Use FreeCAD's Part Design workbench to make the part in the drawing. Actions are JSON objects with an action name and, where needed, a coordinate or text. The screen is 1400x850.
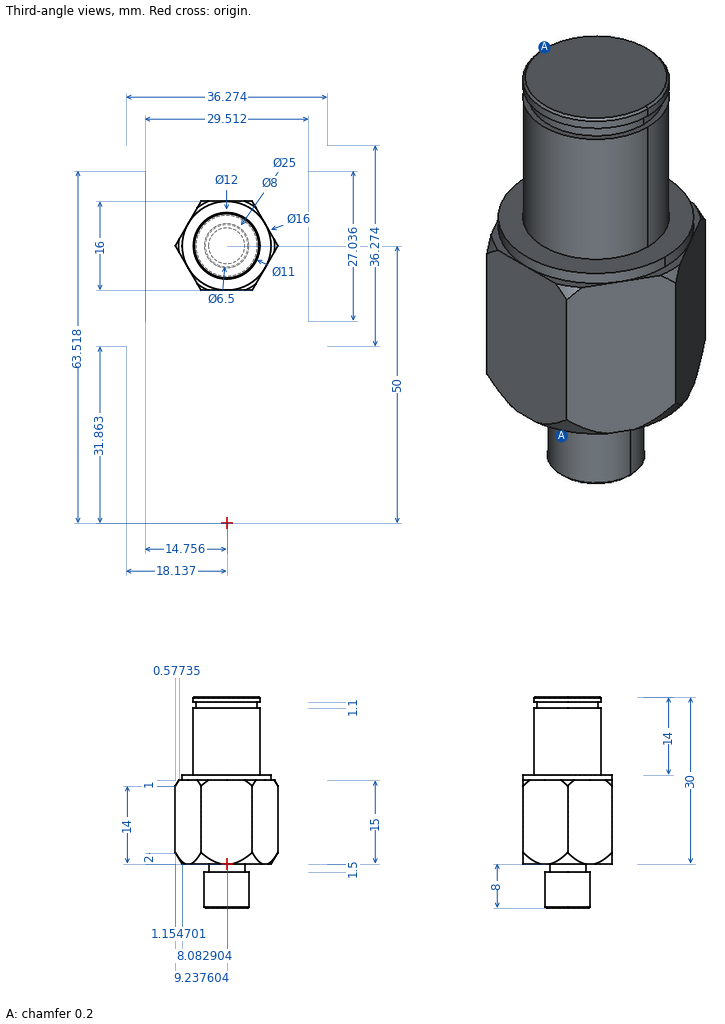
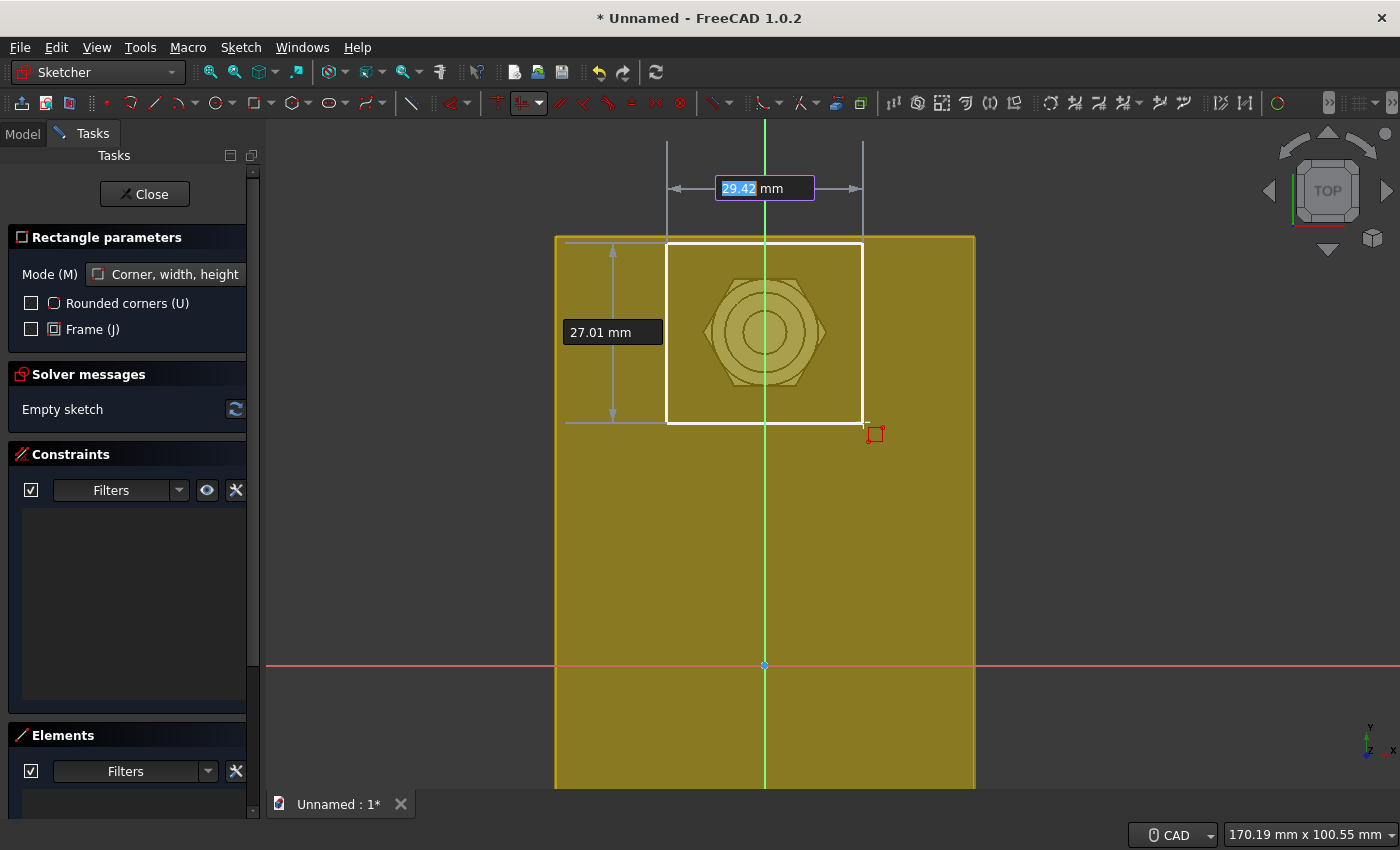
{"action": "type", "text": "29.512"}
{"action": "key", "text": "Tab"}
{"action": "type", "text": "27.036"}
{"action": "key", "text": "Return"}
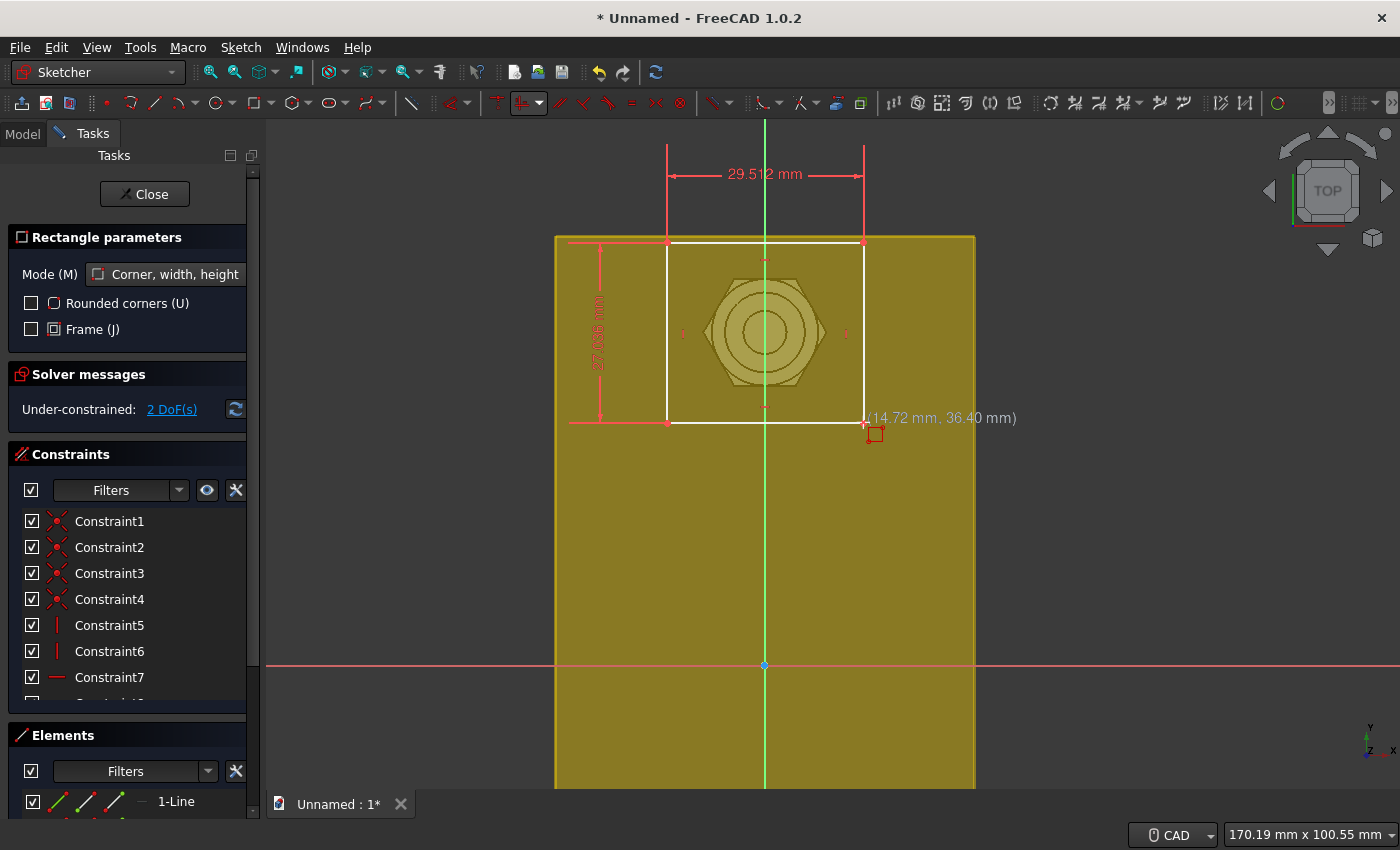
{"action": "left_click", "coordinate": [216, 104]}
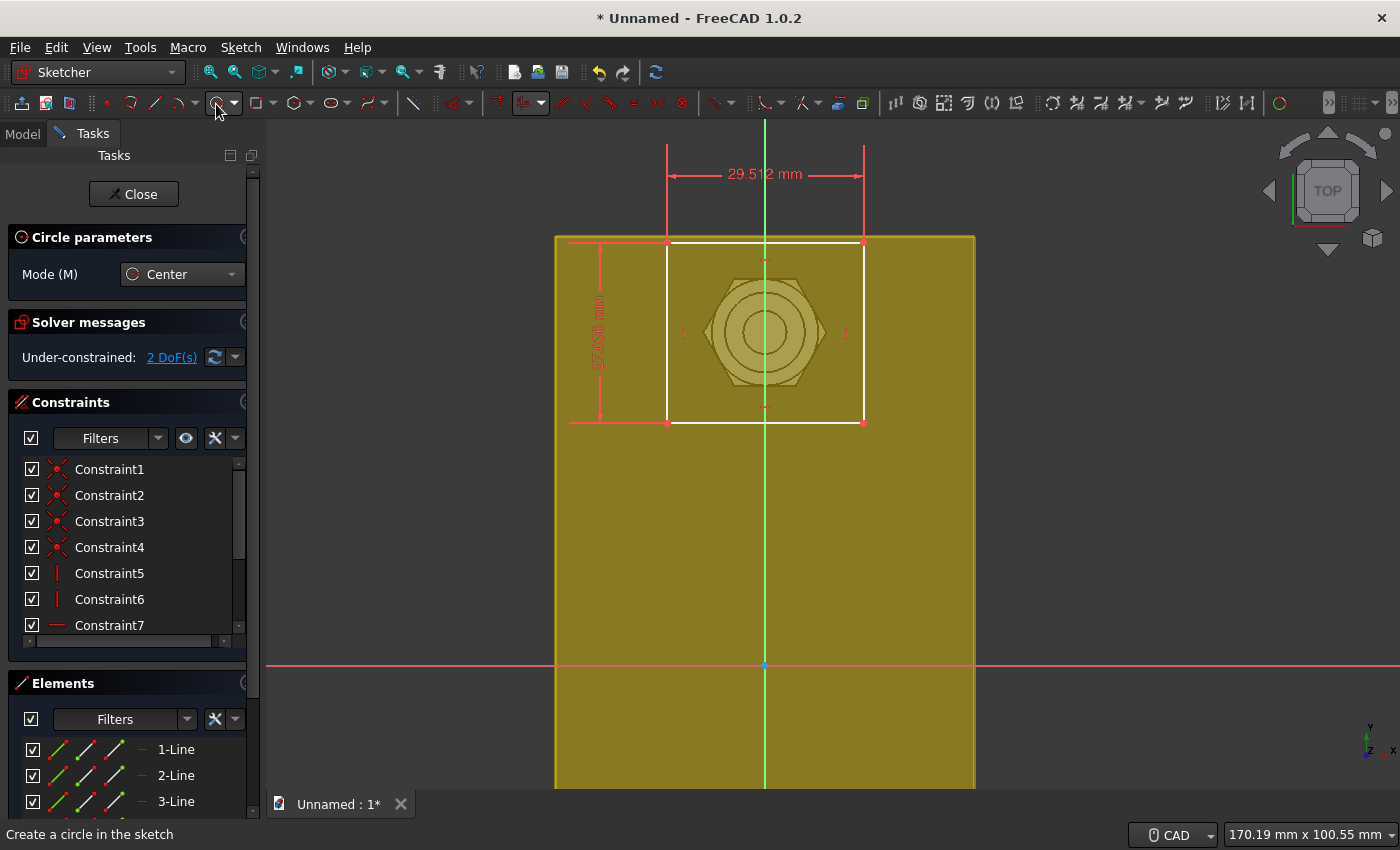
{"action": "left_click", "coordinate": [765, 332]}
{"action": "mouse_move", "coordinate": [791, 306]}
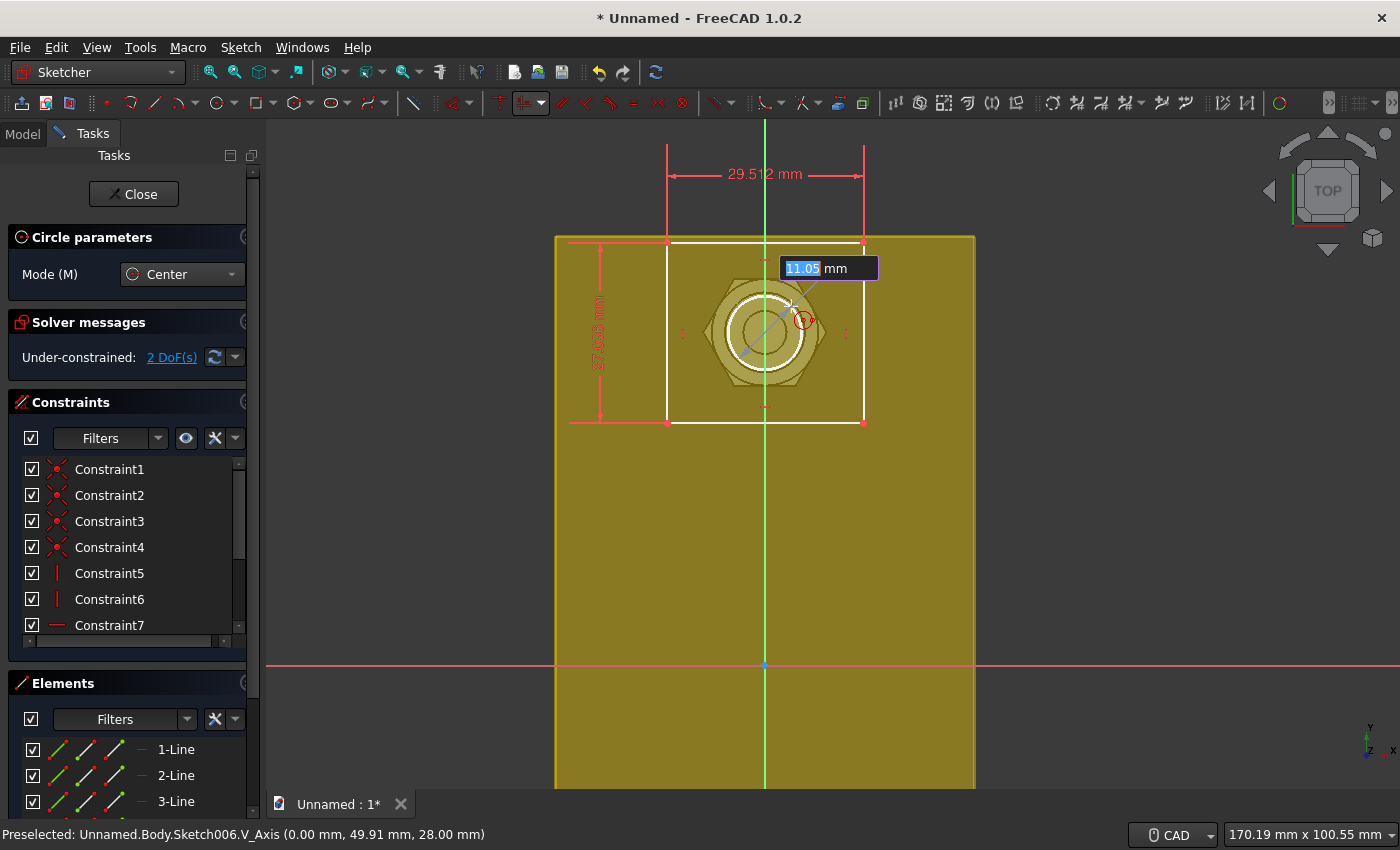
{"action": "type", "text": "11"}
{"action": "key", "text": "Return"}
{"action": "key", "text": "Escape"}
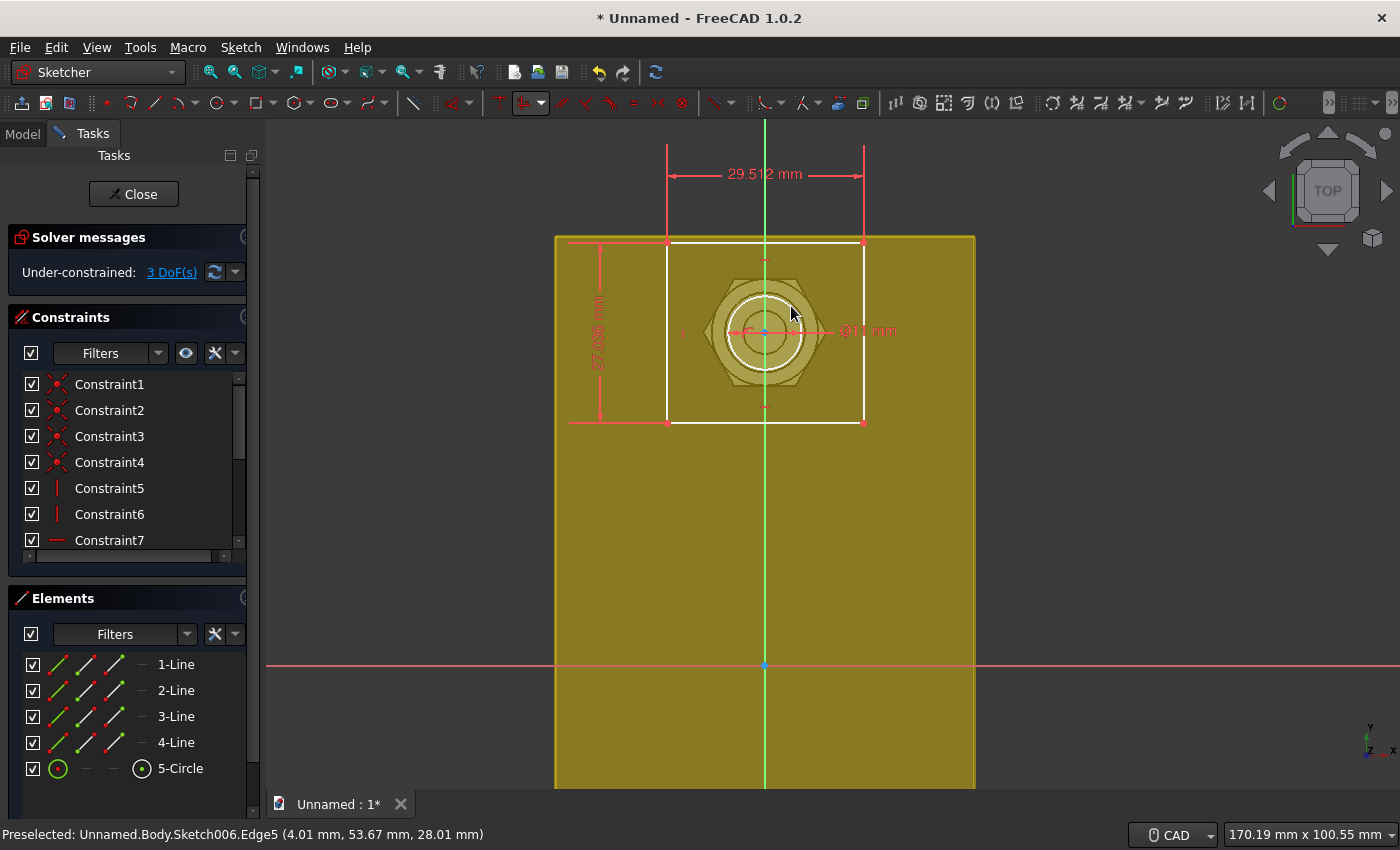
{"action": "left_click", "coordinate": [452, 104]}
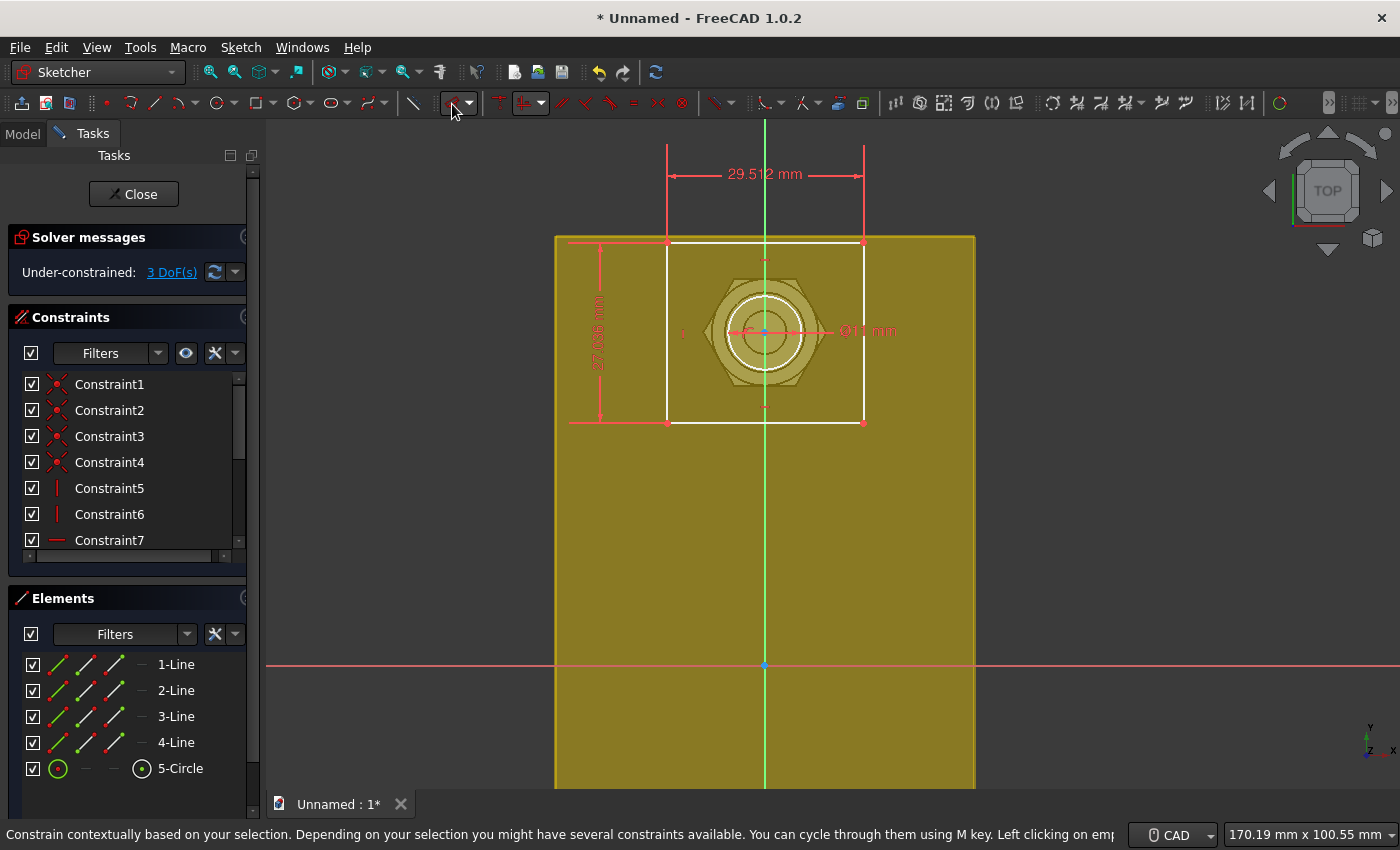
{"action": "left_click", "coordinate": [765, 333]}
{"action": "left_click", "coordinate": [799, 499]}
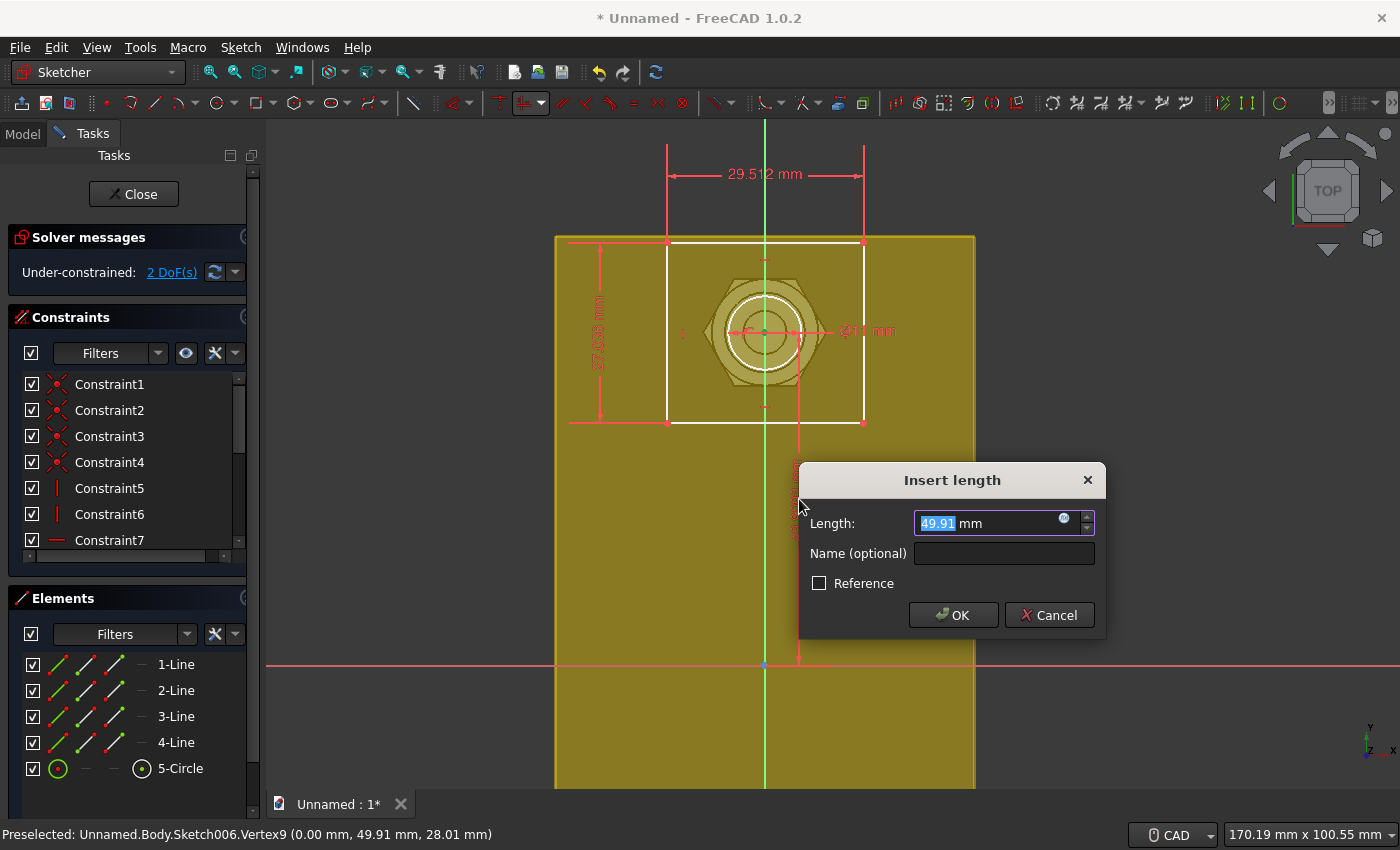
{"action": "type", "text": "50"}
{"action": "key", "text": "Return"}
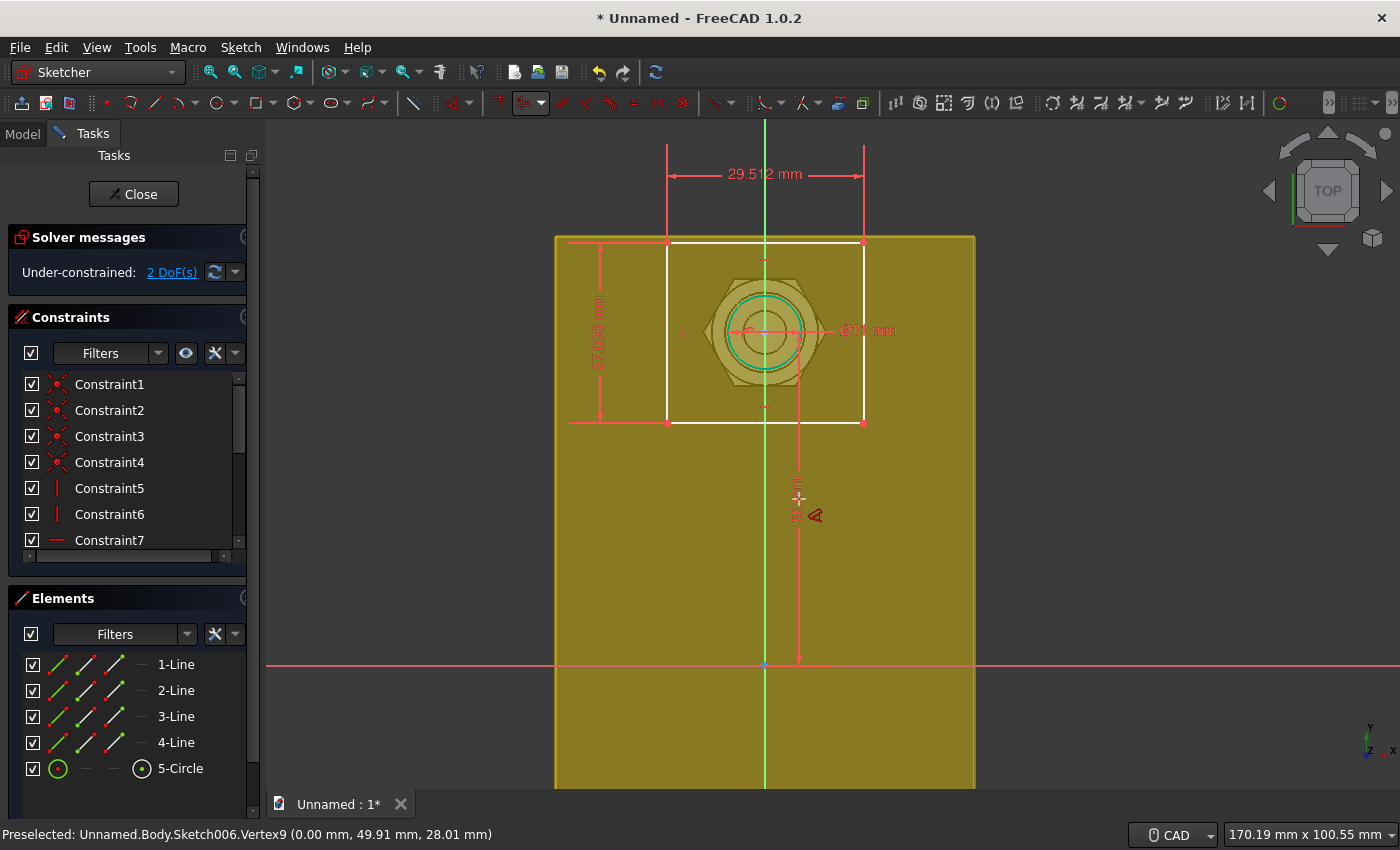
{"action": "left_click", "coordinate": [667, 243]}
{"action": "left_click", "coordinate": [716, 700]}